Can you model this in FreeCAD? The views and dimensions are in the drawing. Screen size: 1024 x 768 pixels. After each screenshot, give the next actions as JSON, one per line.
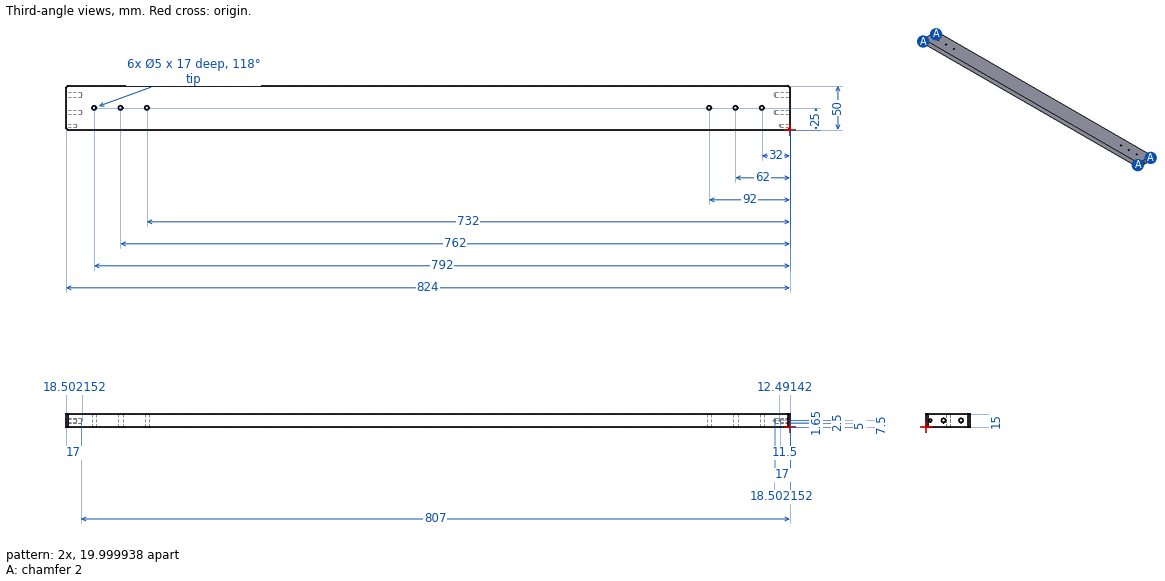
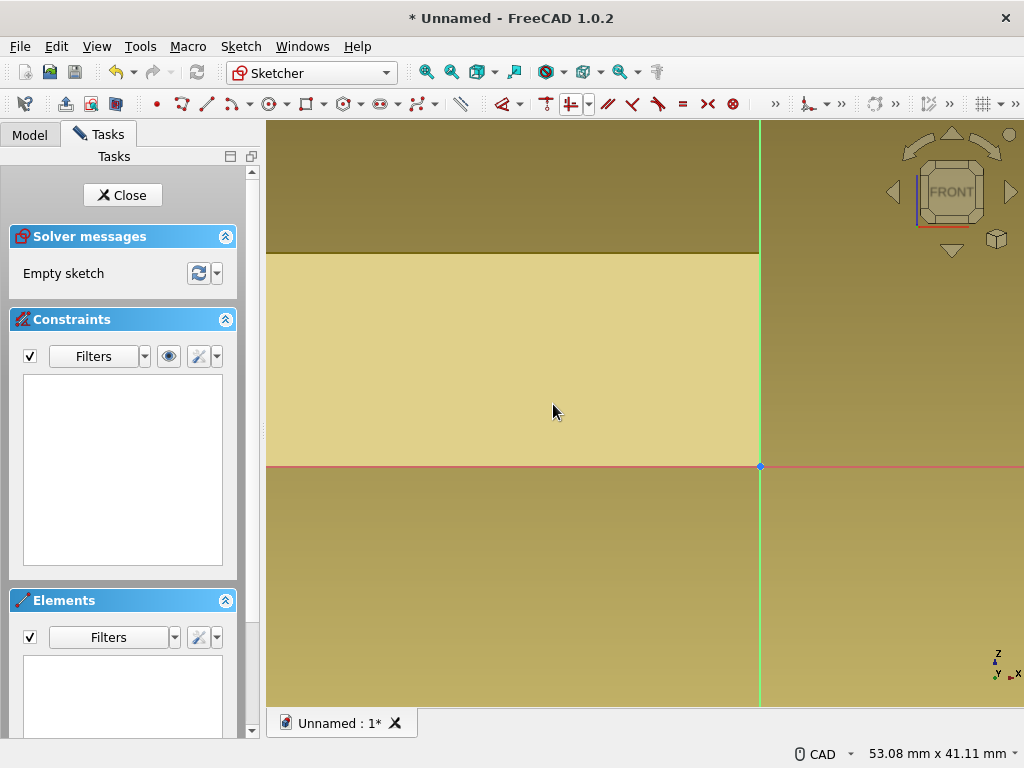
{"action": "left_click", "coordinate": [182, 104]}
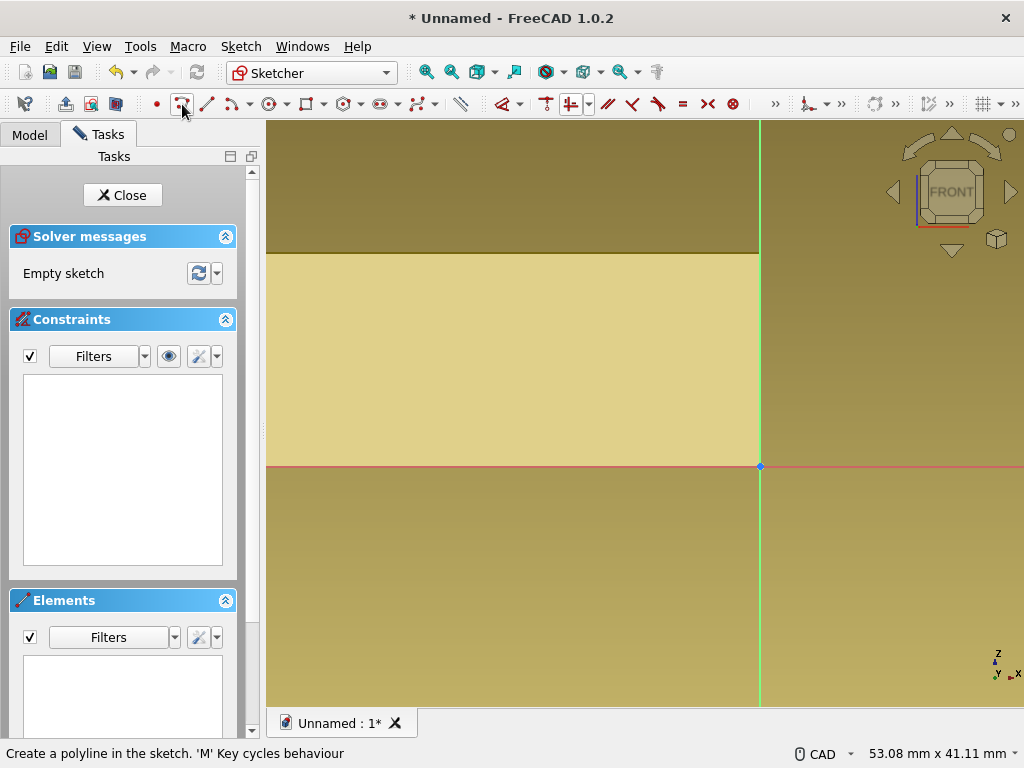
{"action": "left_click", "coordinate": [760, 395]}
{"action": "left_click", "coordinate": [517, 395]}
{"action": "left_click", "coordinate": [496, 360]}
{"action": "left_click", "coordinate": [751, 360]}
{"action": "left_click", "coordinate": [760, 396]}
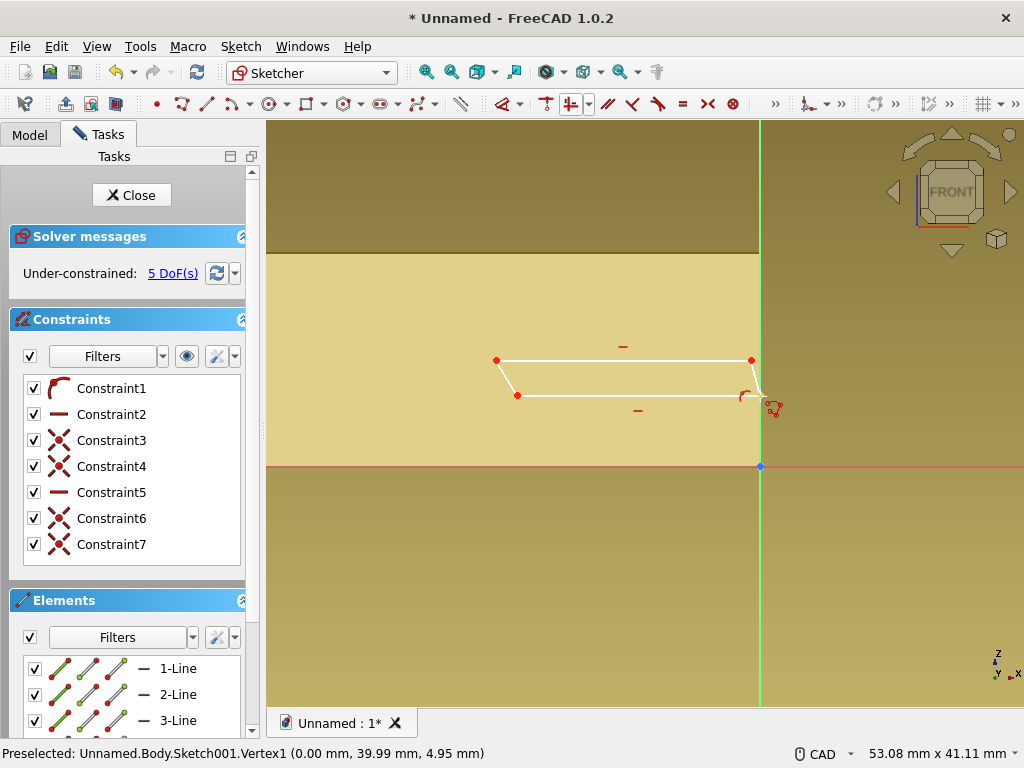
{"action": "left_click", "coordinate": [207, 104]}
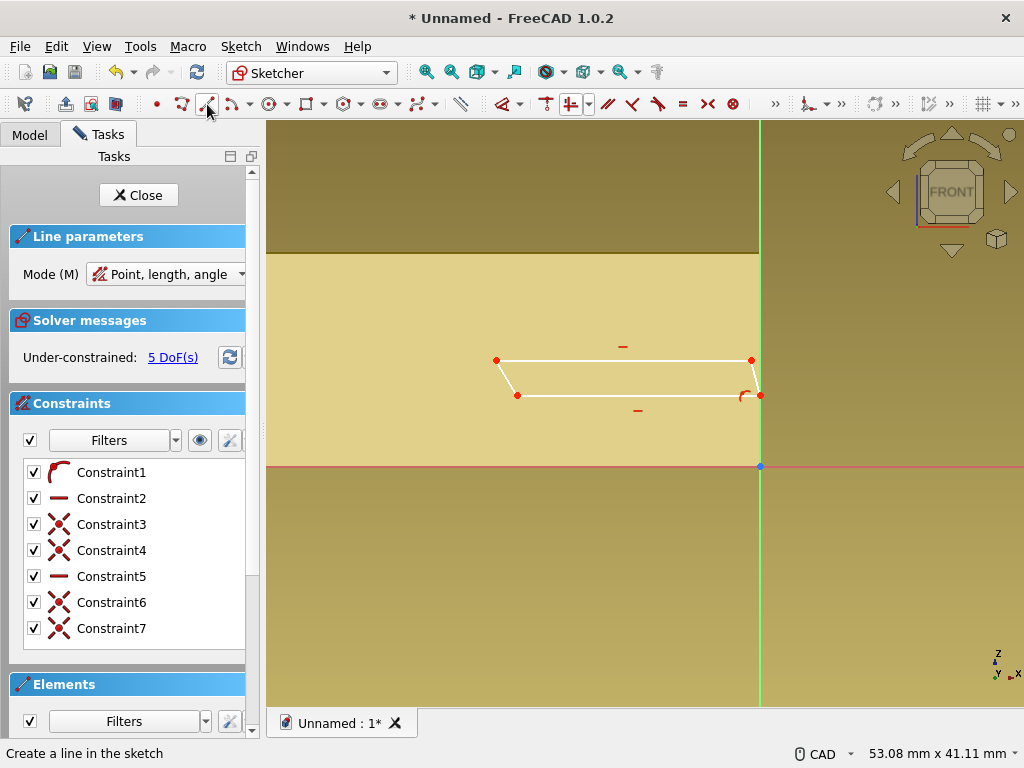
{"action": "left_click", "coordinate": [469, 360]}
{"action": "left_click", "coordinate": [390, 360]}
{"action": "key", "text": "Escape"}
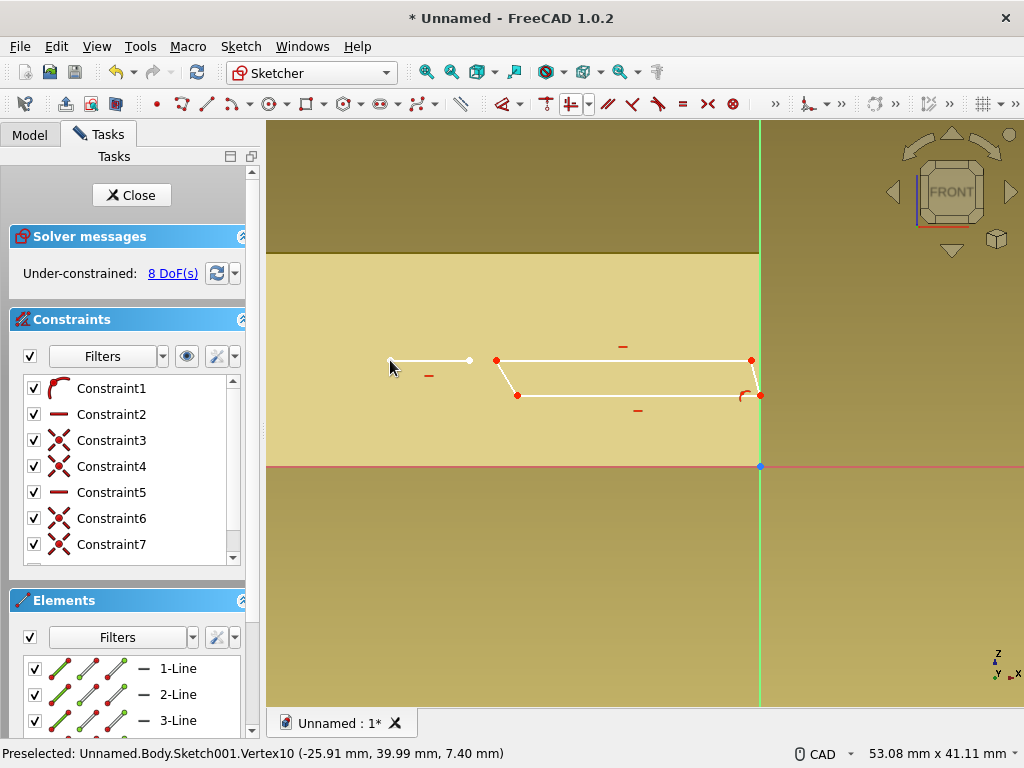
{"action": "left_click", "coordinate": [445, 361]}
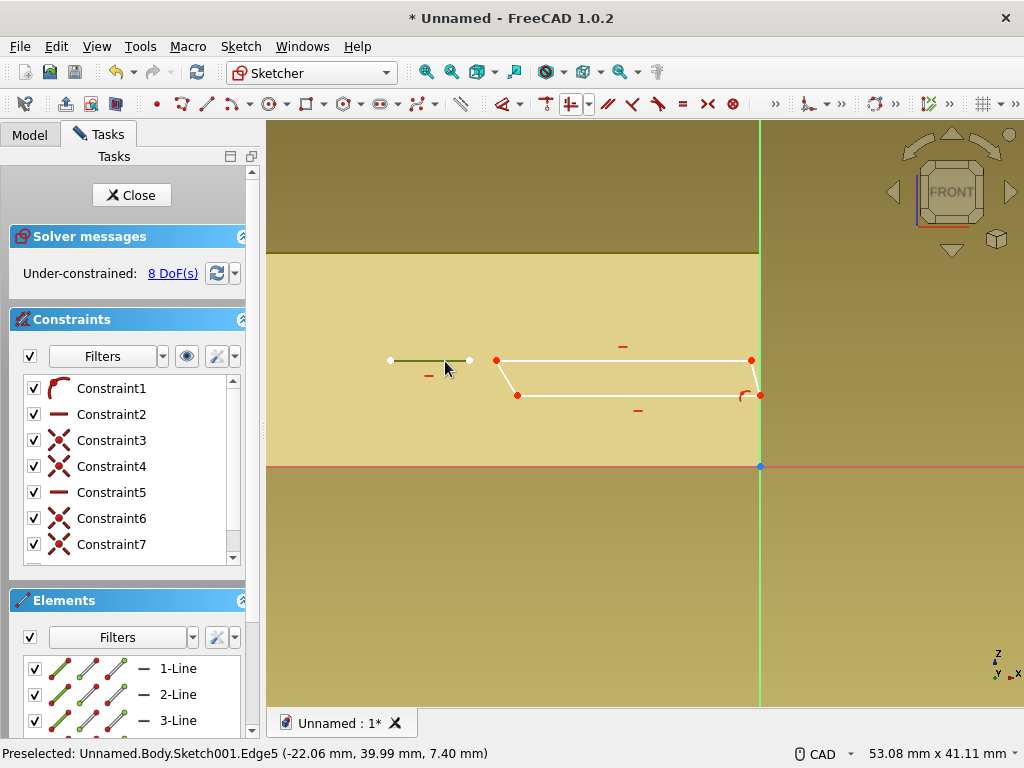
{"action": "left_click", "coordinate": [461, 104]}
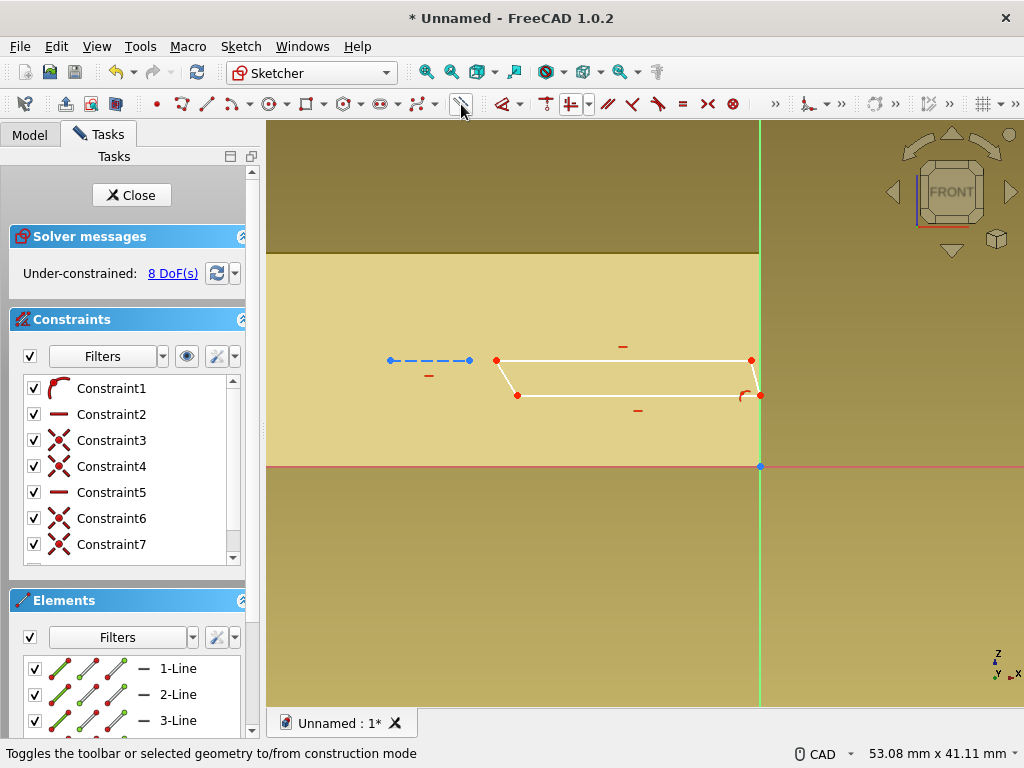
{"action": "scroll", "coordinate": [757, 385], "scroll_direction": "up", "scroll_amount": 2}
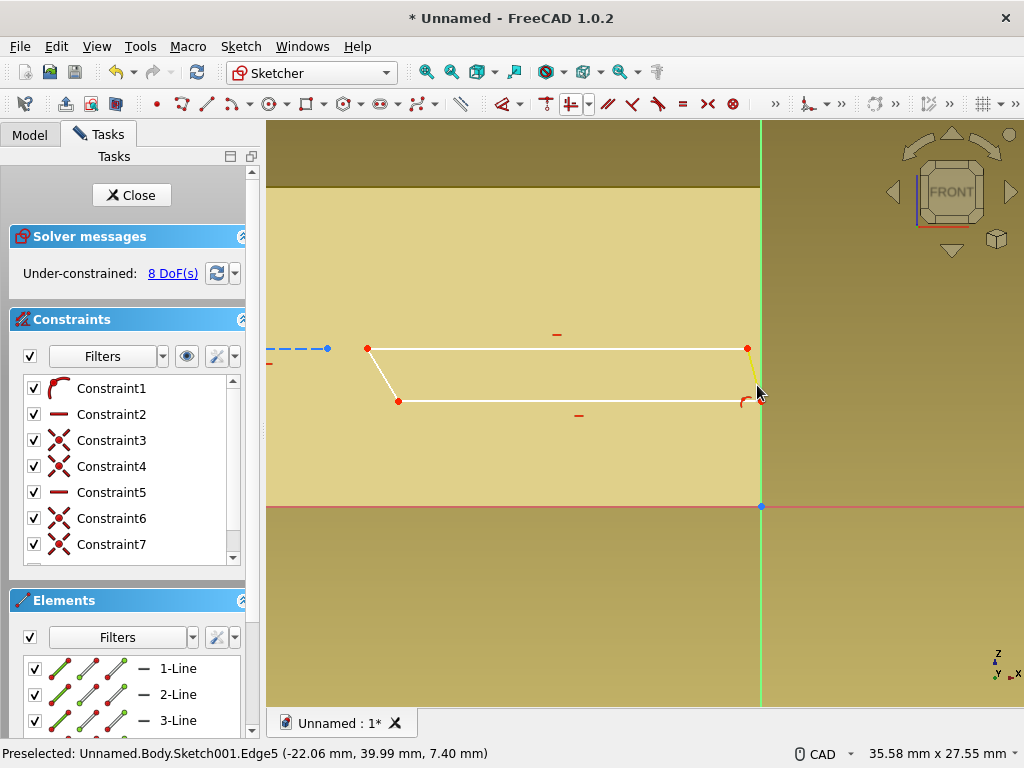
{"action": "left_click", "coordinate": [757, 386]}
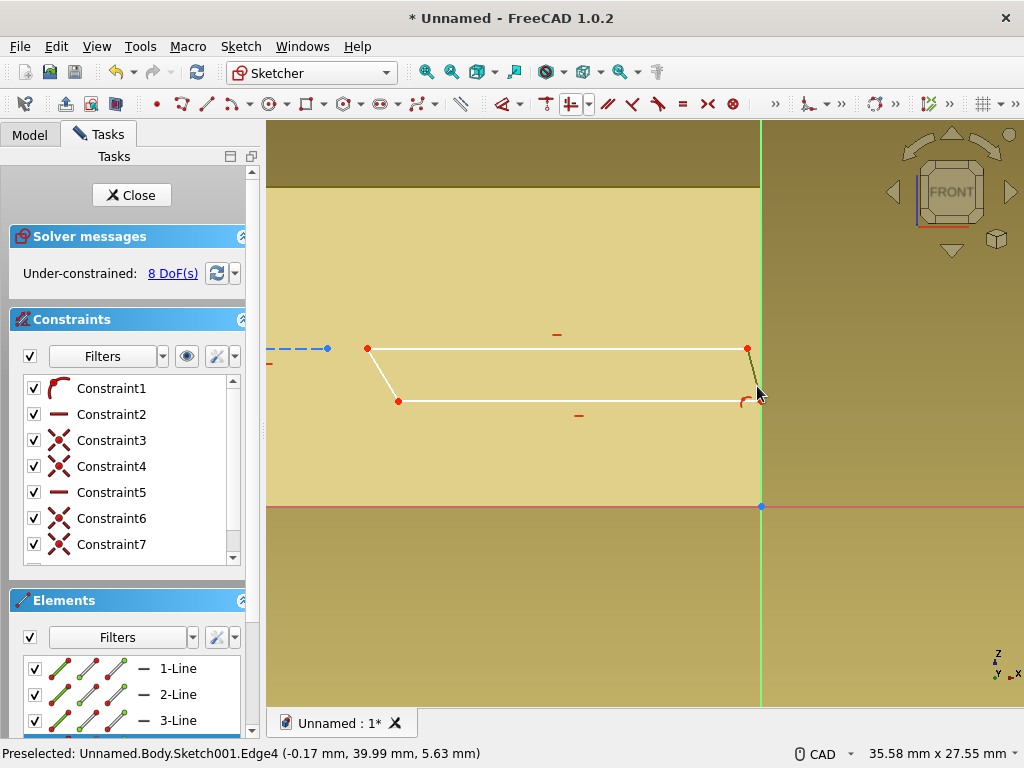
{"action": "key", "text": "v"}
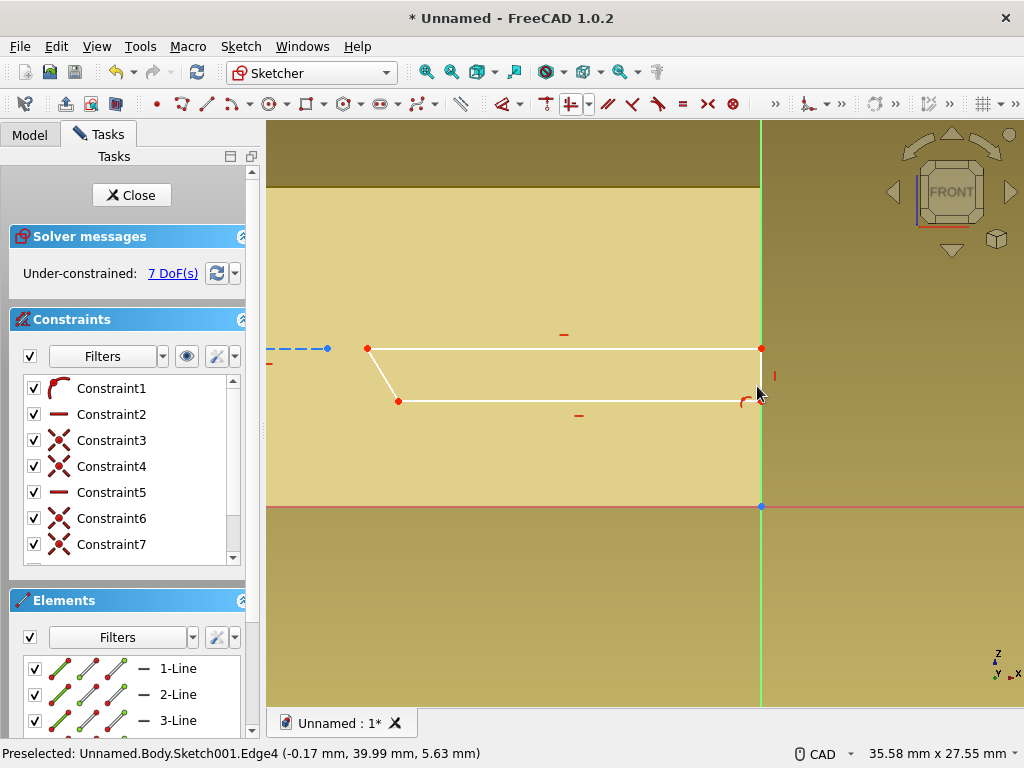
{"action": "left_click", "coordinate": [502, 104]}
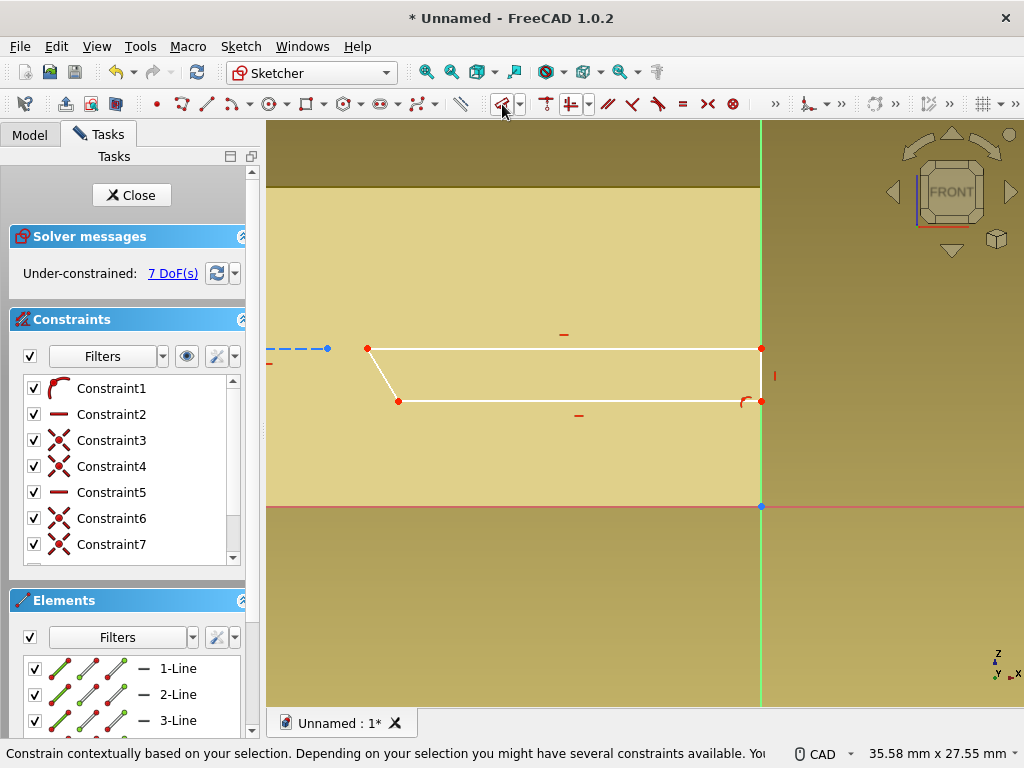
{"action": "left_click", "coordinate": [652, 401]}
{"action": "left_click", "coordinate": [580, 367]}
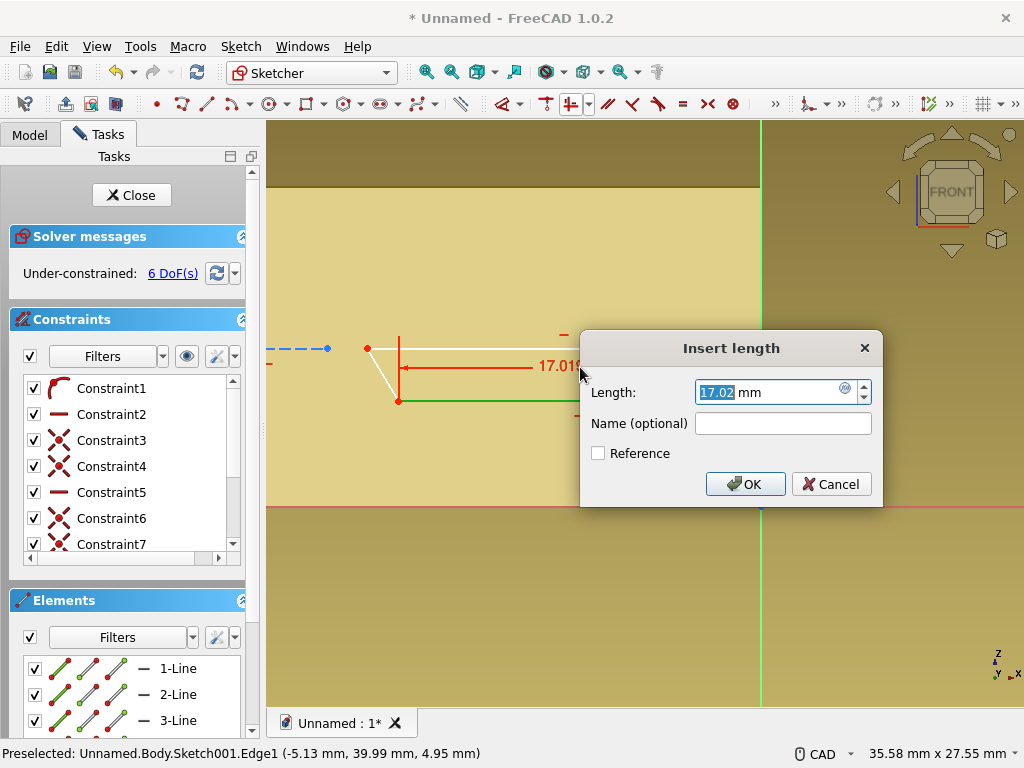
{"action": "type", "text": "17"}
{"action": "key", "text": "Return"}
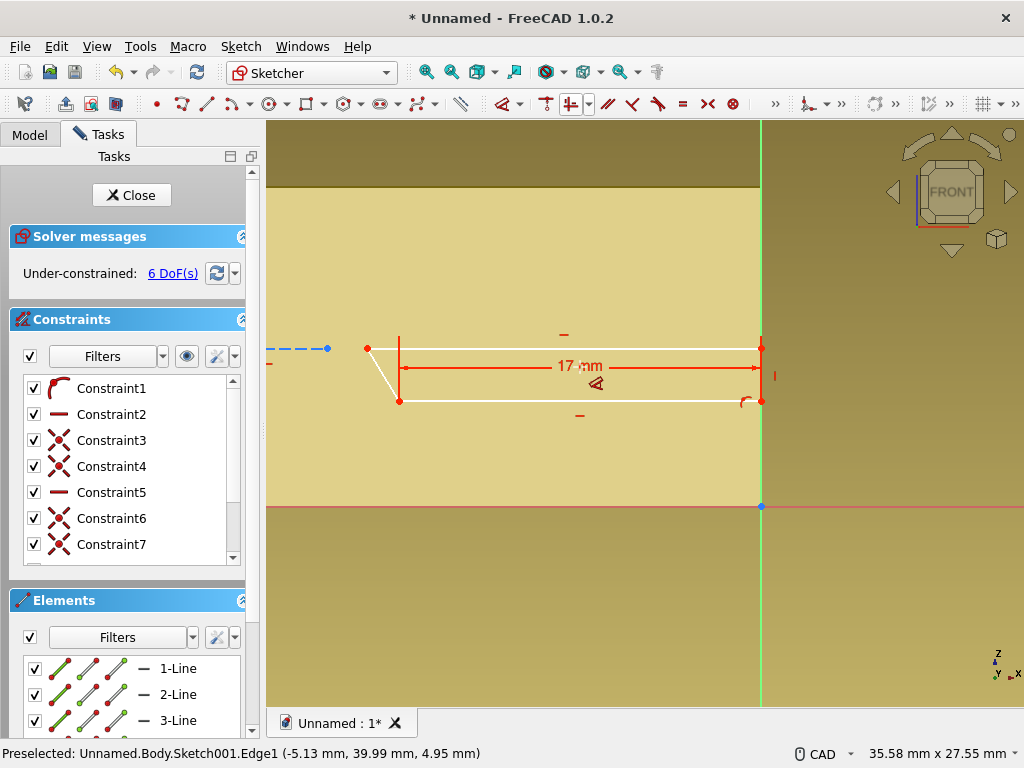
{"action": "left_click", "coordinate": [761, 401]}
{"action": "left_click", "coordinate": [795, 454]}